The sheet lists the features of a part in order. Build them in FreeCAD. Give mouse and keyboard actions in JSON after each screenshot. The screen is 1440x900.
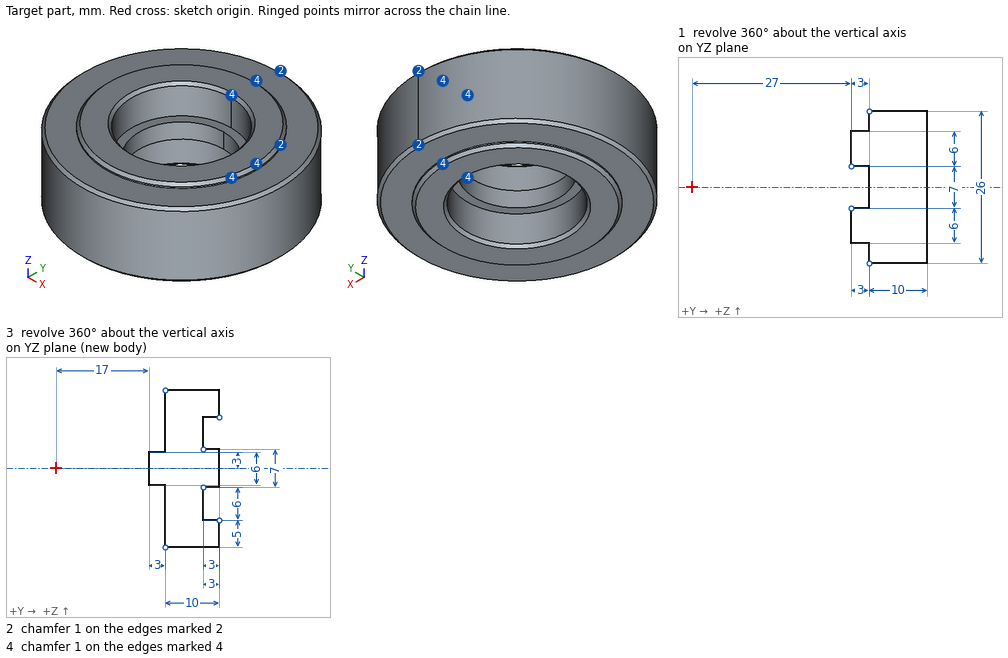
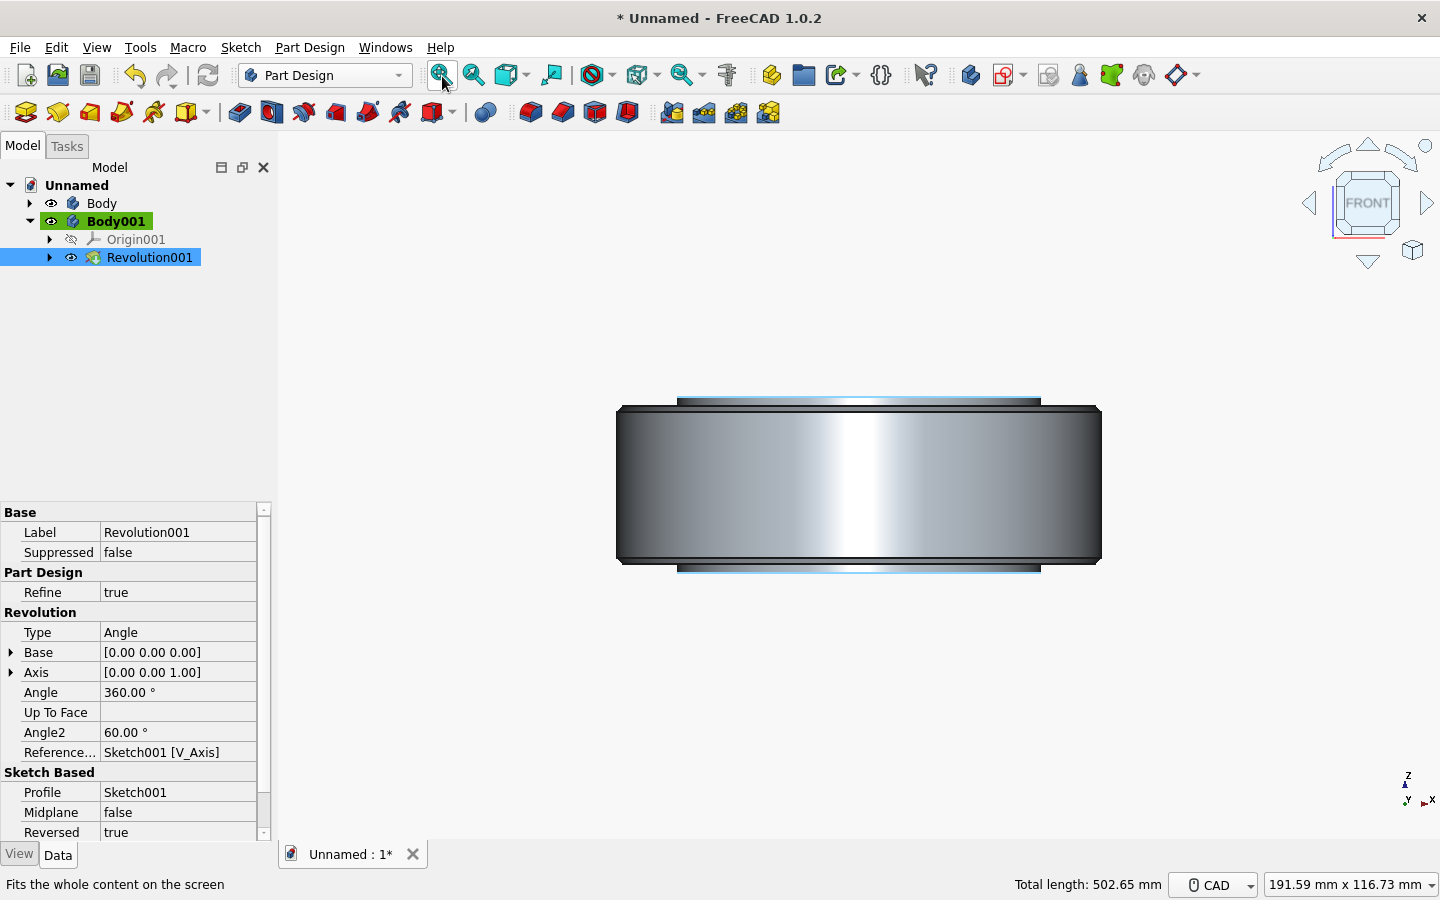
{"action": "key", "text": "3"}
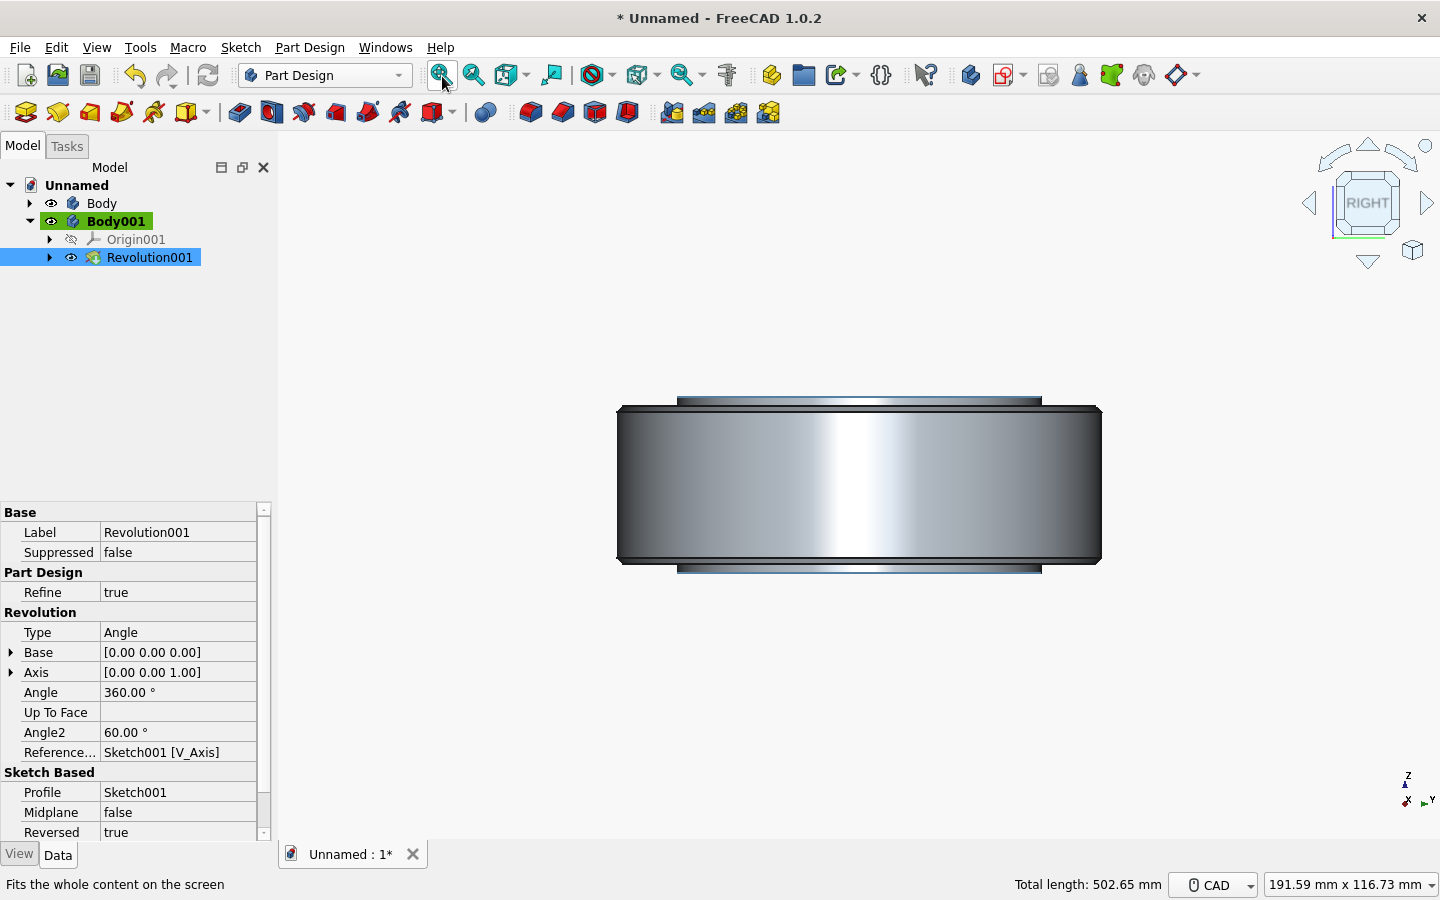
{"action": "left_click", "coordinate": [442, 76]}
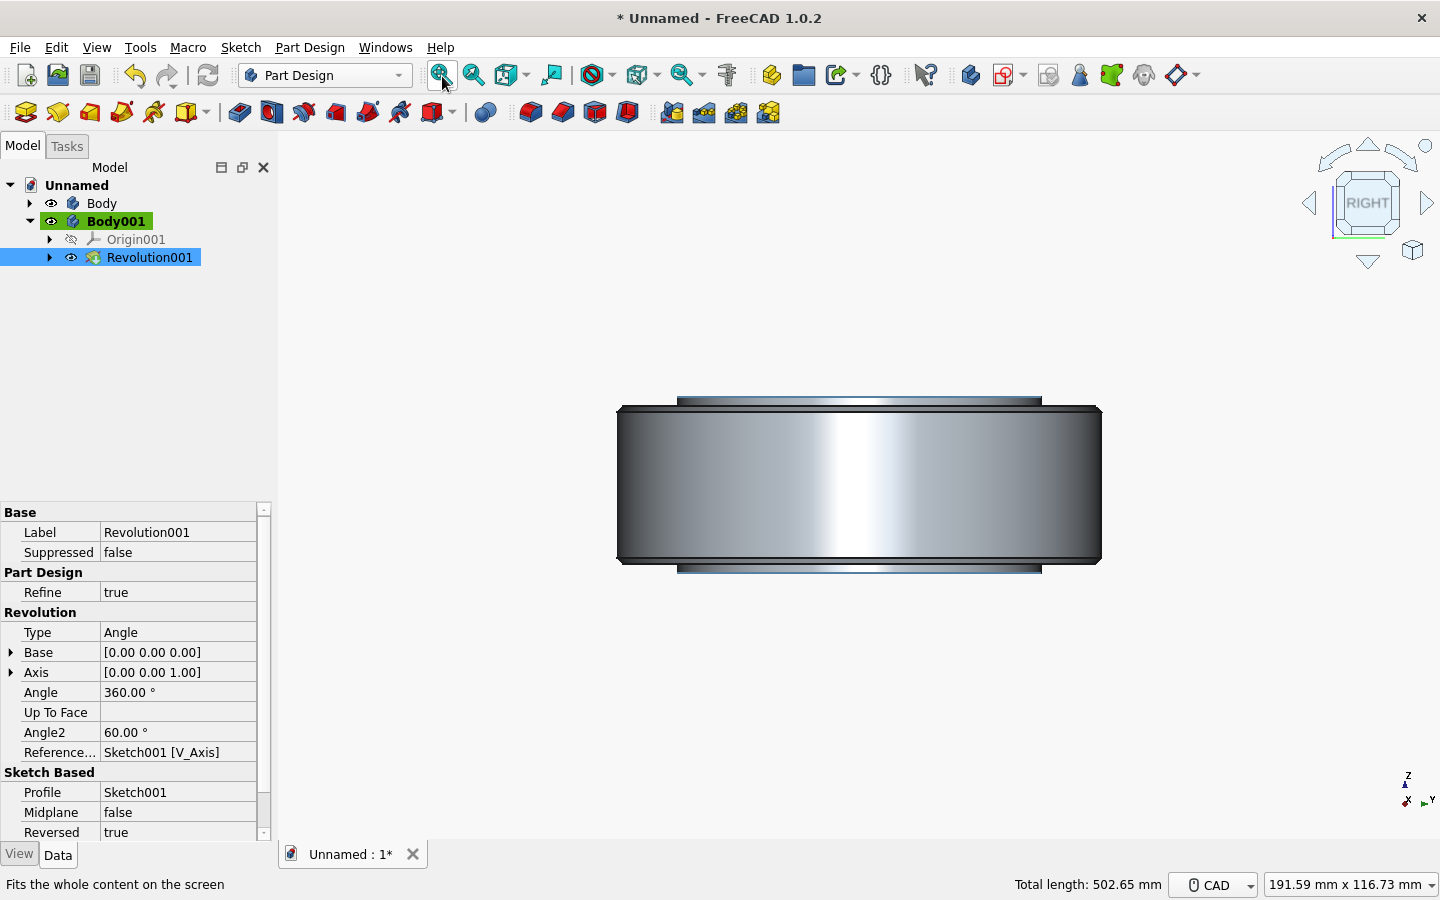
{"action": "key", "text": "5"}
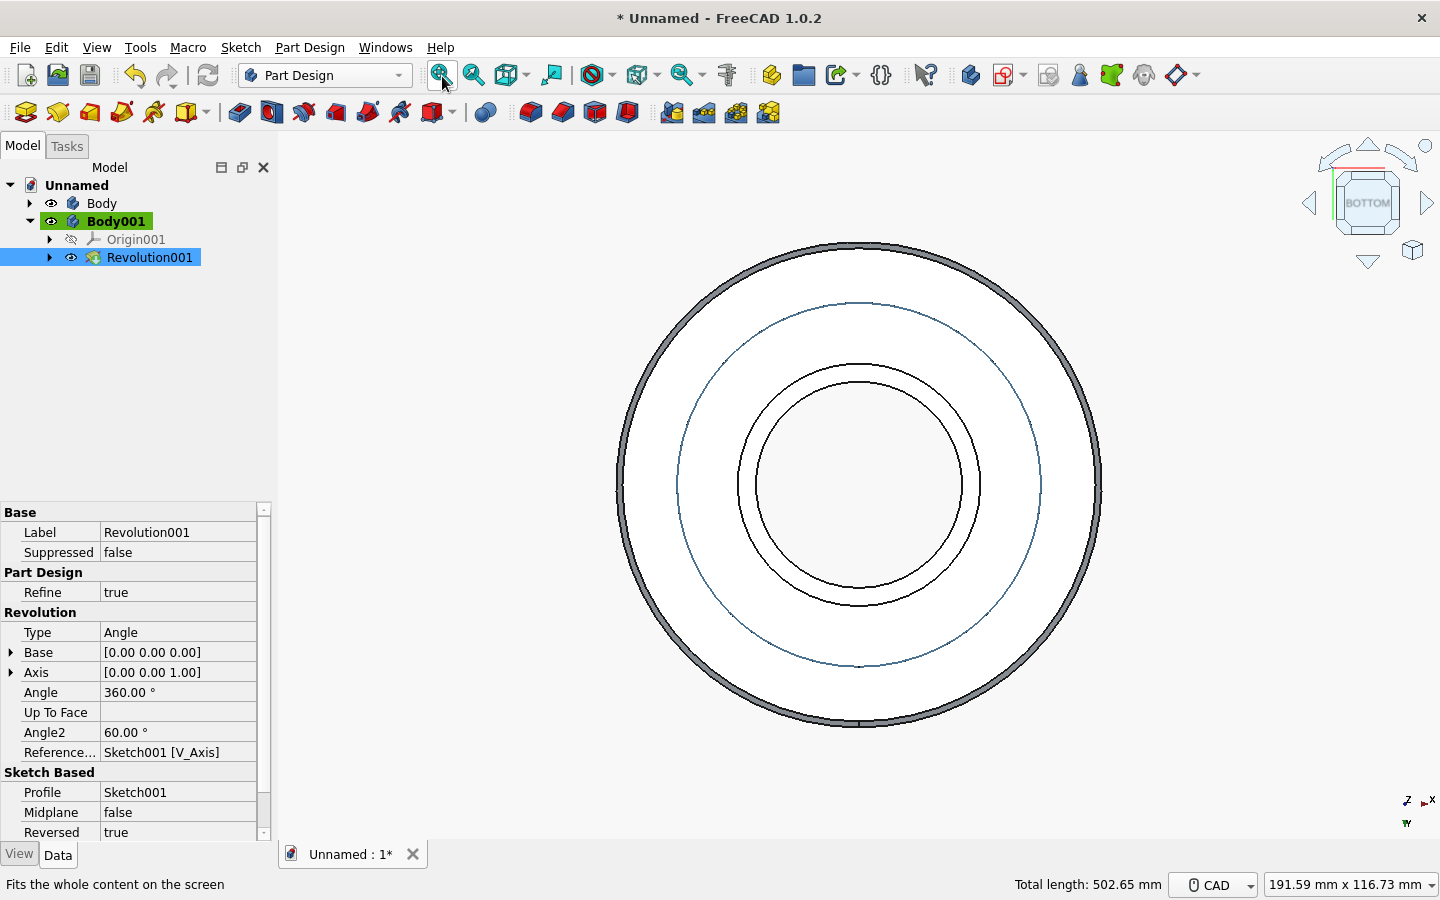
{"action": "left_click", "coordinate": [859, 363], "text": "ctrl"}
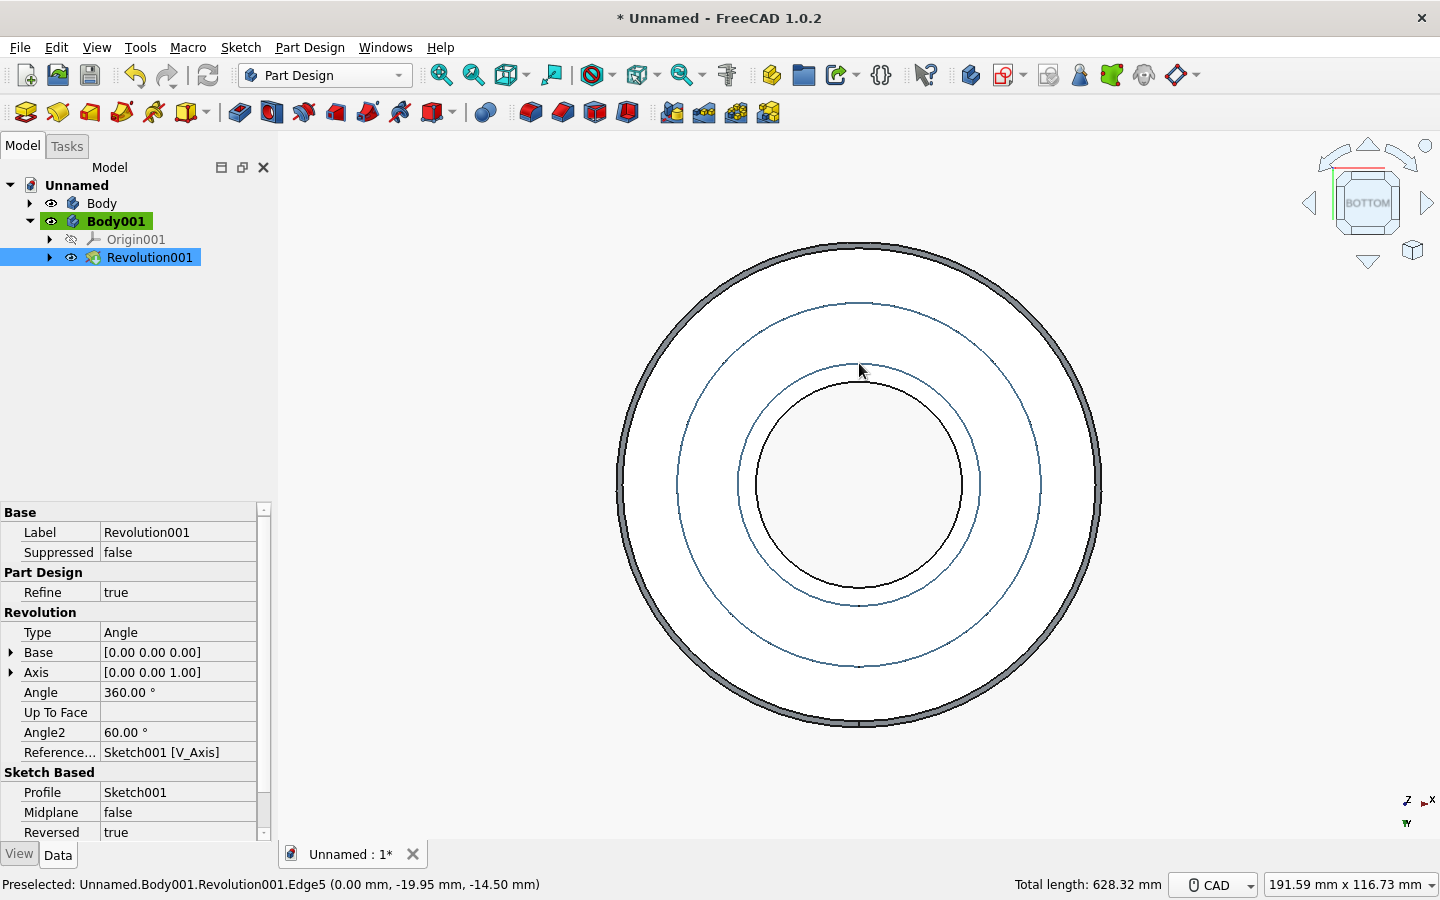
{"action": "left_click", "coordinate": [564, 112]}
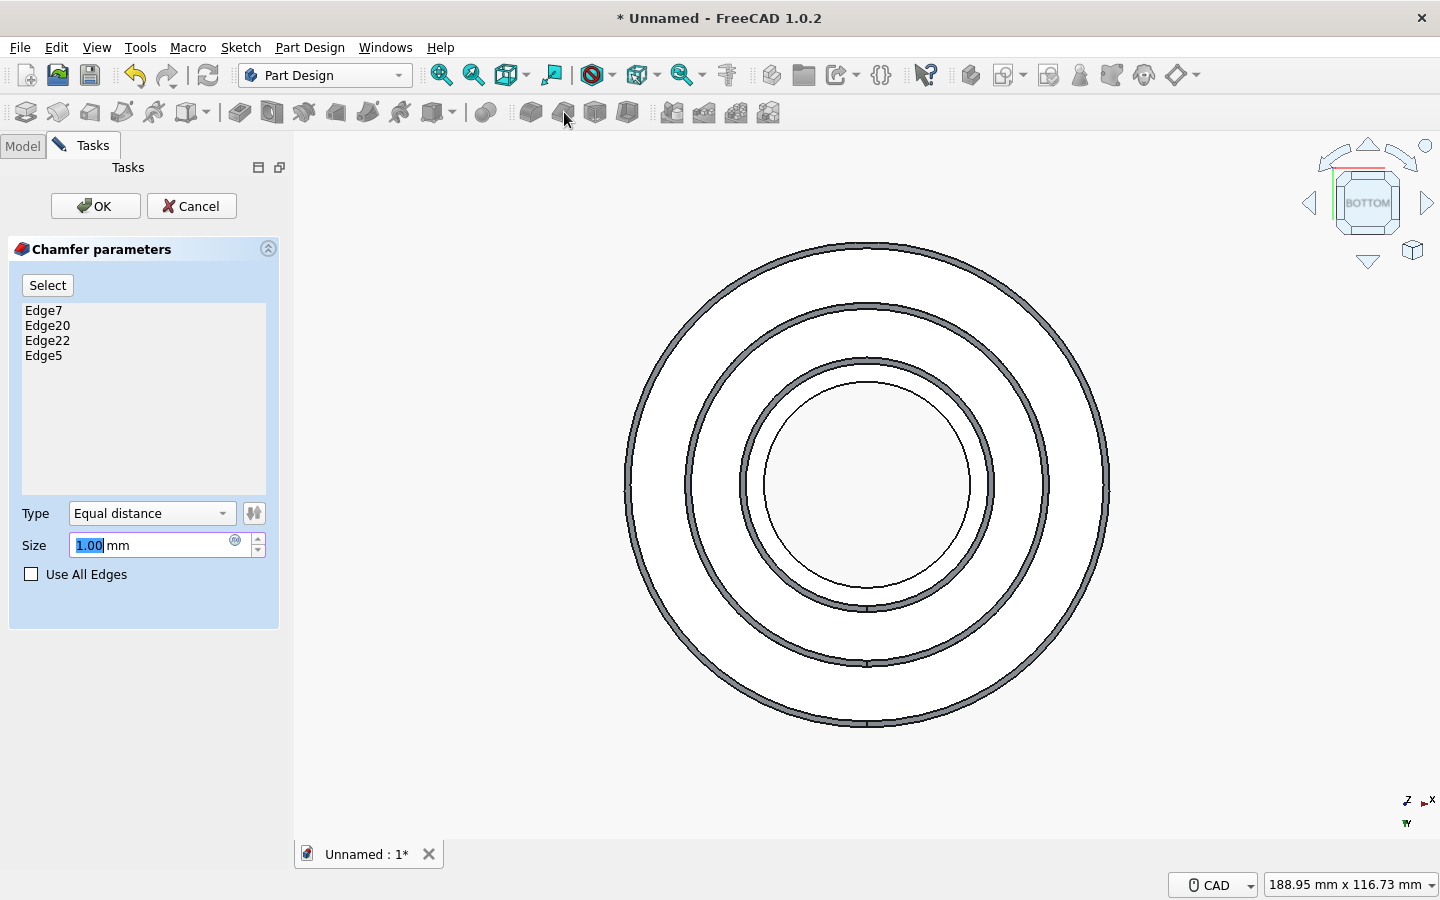
{"action": "type", "text": "1"}
{"action": "key", "text": "Tab"}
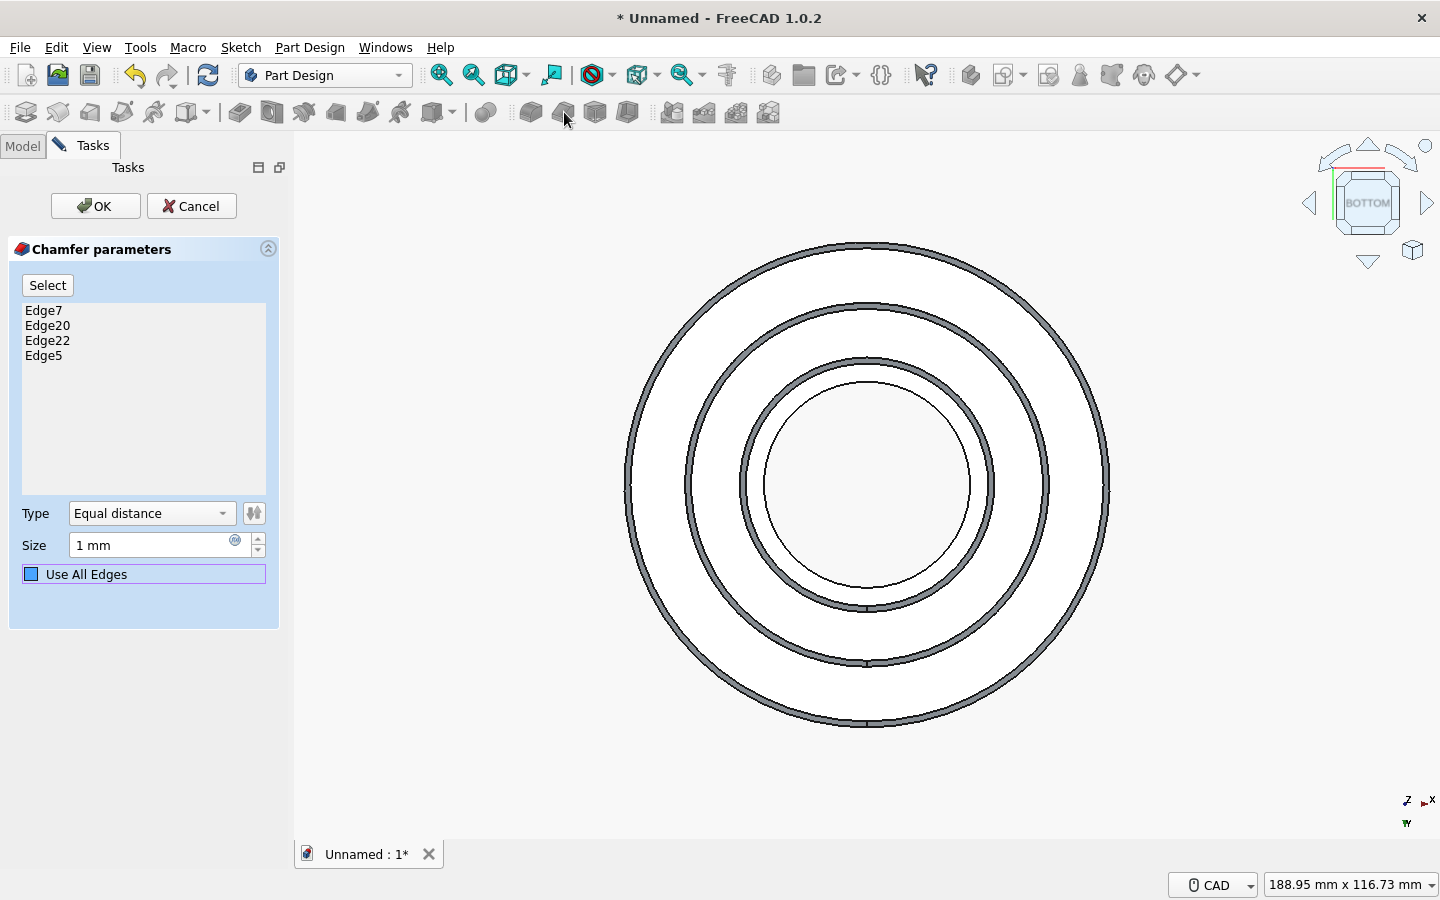
{"action": "left_click", "coordinate": [96, 206]}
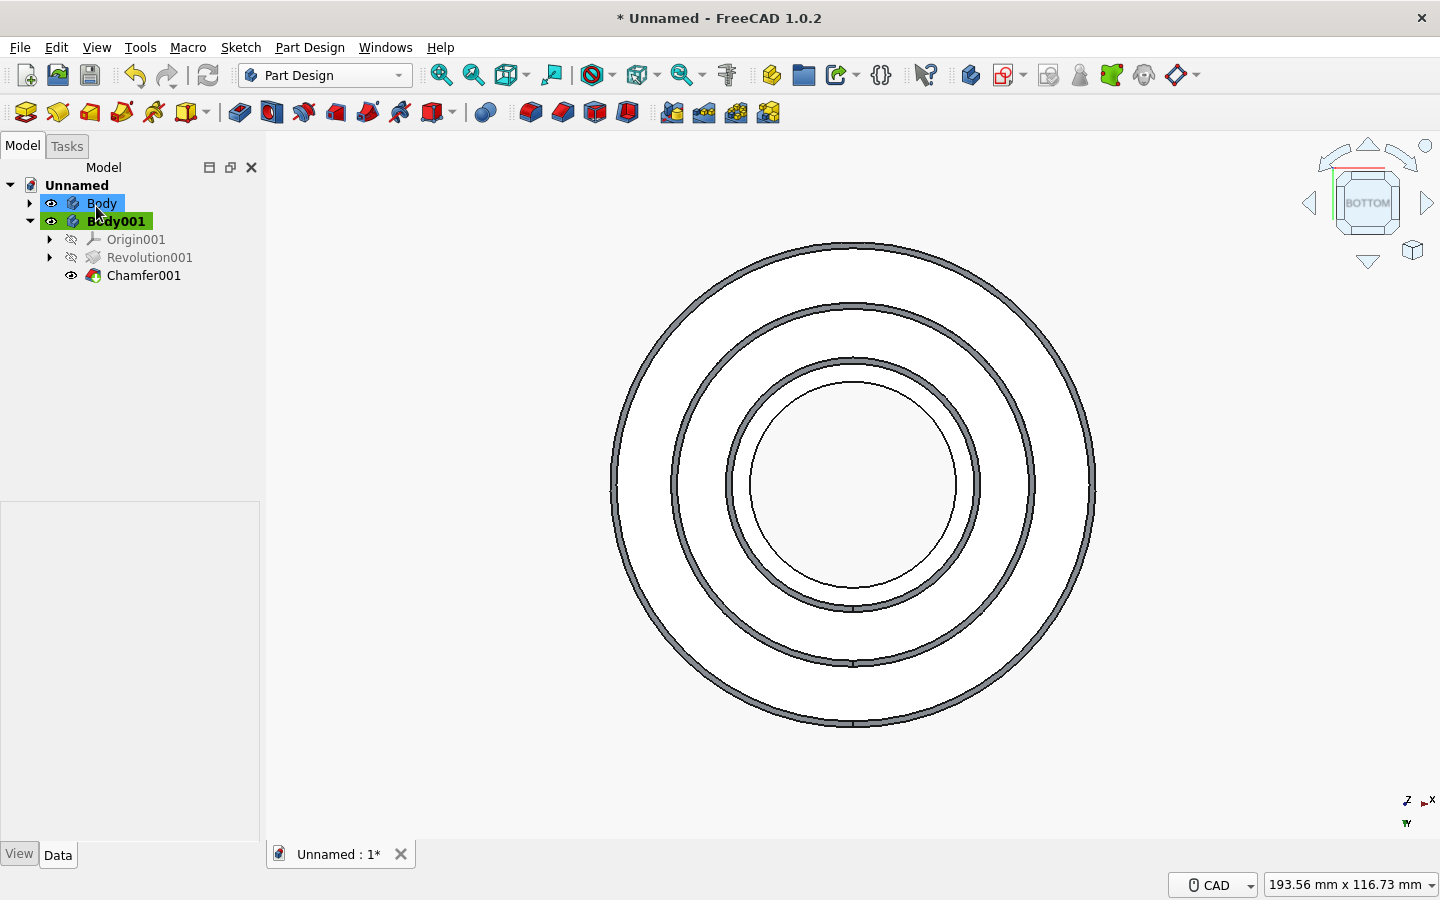
{"action": "key", "text": "0"}